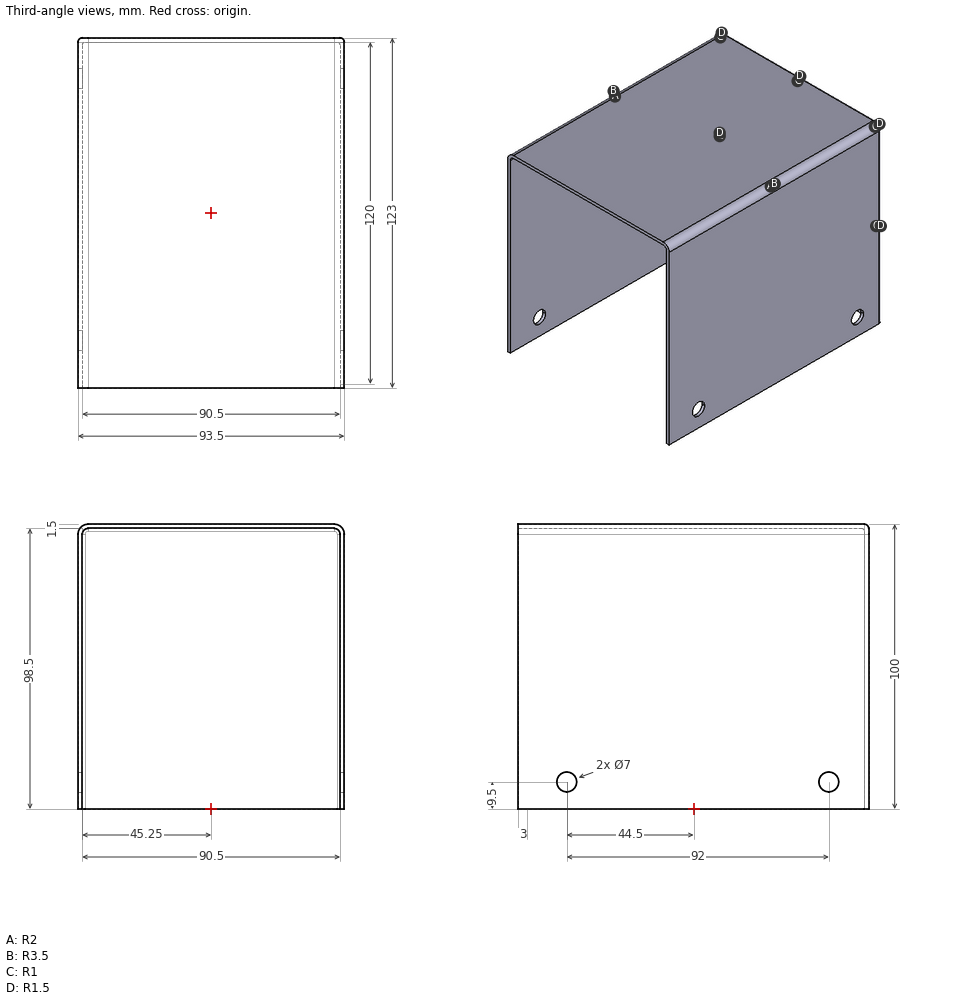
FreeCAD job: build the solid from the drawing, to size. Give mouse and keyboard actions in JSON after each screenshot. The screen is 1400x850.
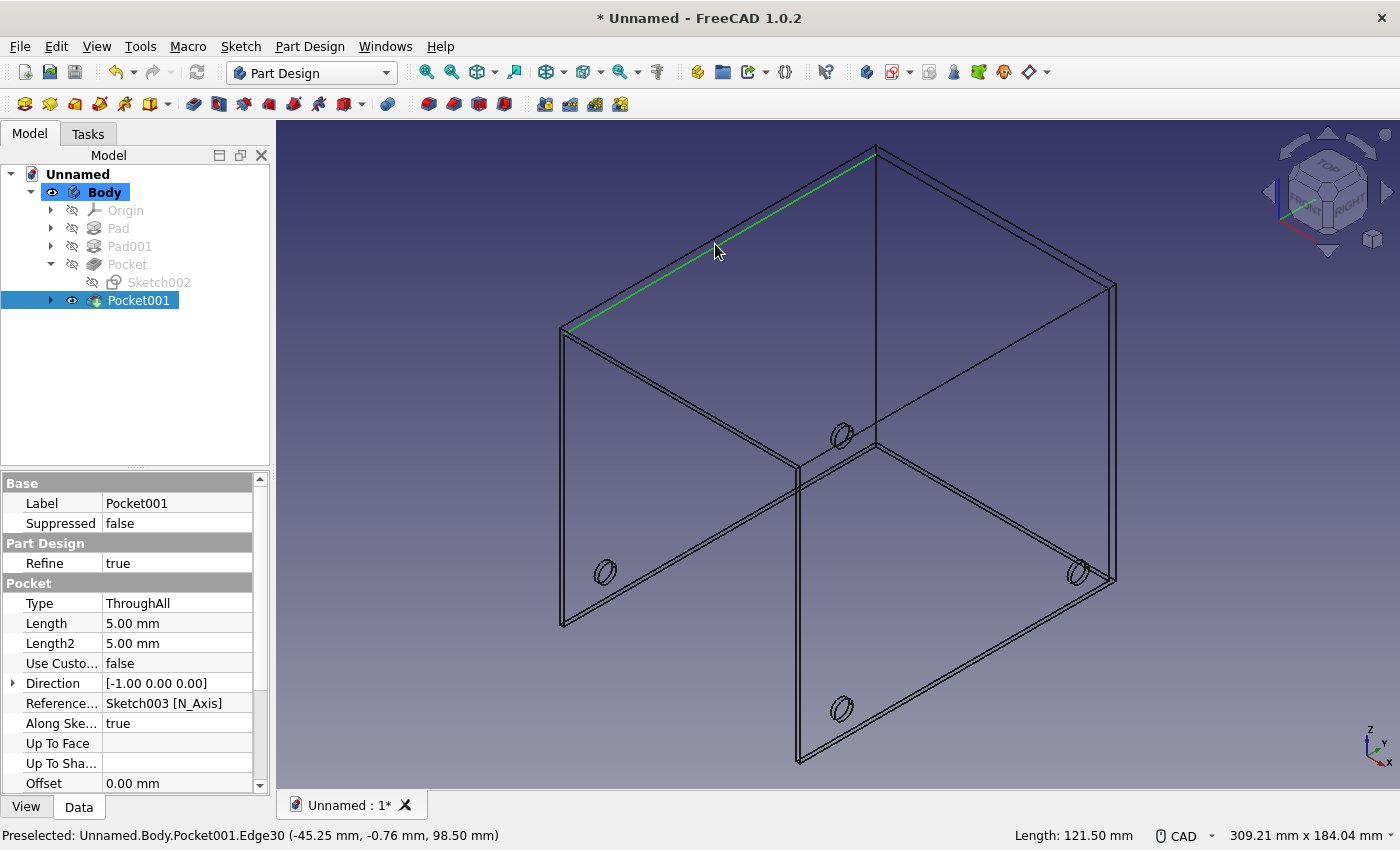
{"action": "scroll", "coordinate": [952, 378], "scroll_direction": "up", "scroll_amount": 6}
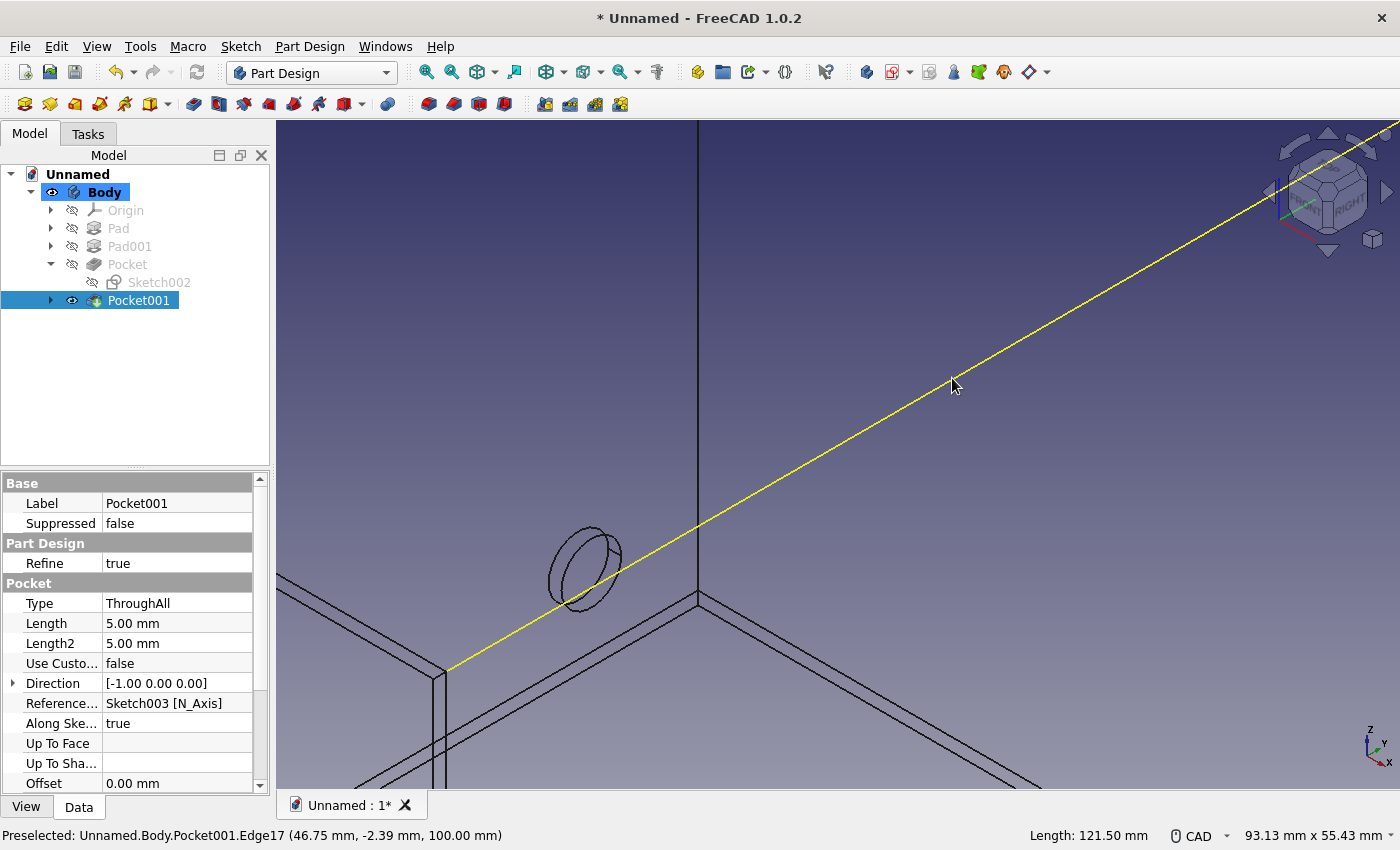
{"action": "left_click", "coordinate": [427, 72]}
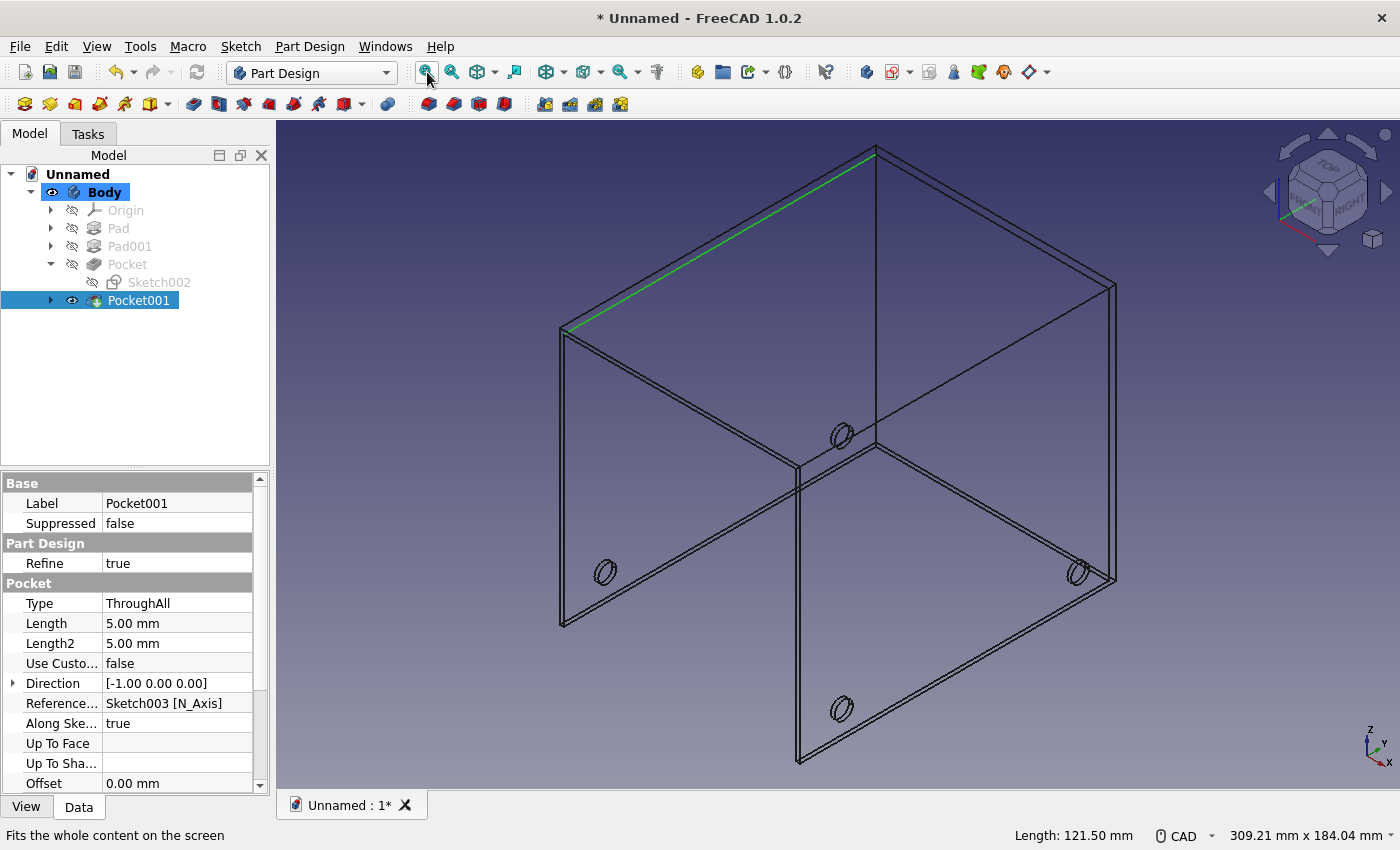
{"action": "key", "text": "2"}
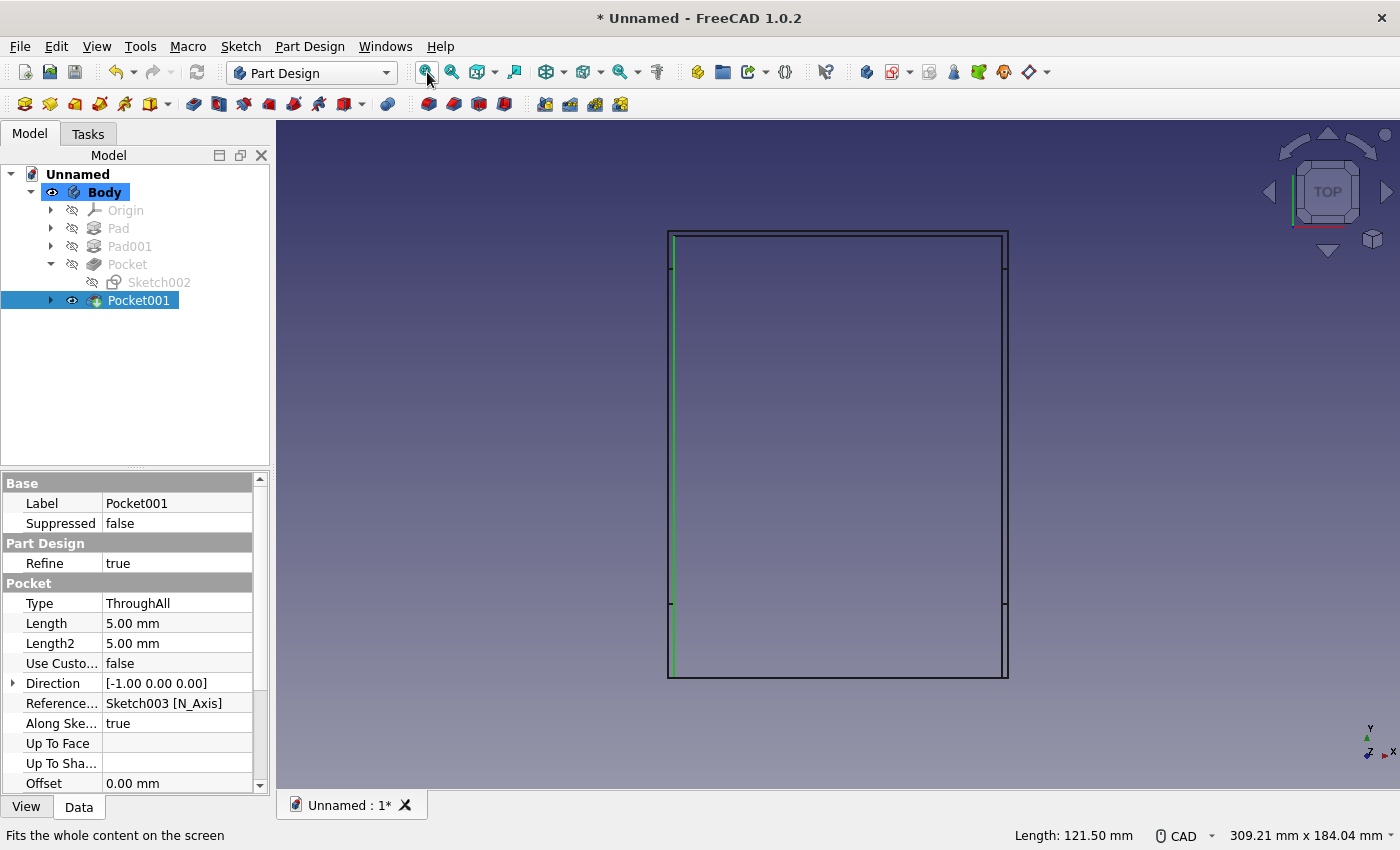
{"action": "scroll", "coordinate": [1002, 456], "scroll_direction": "up", "scroll_amount": 6}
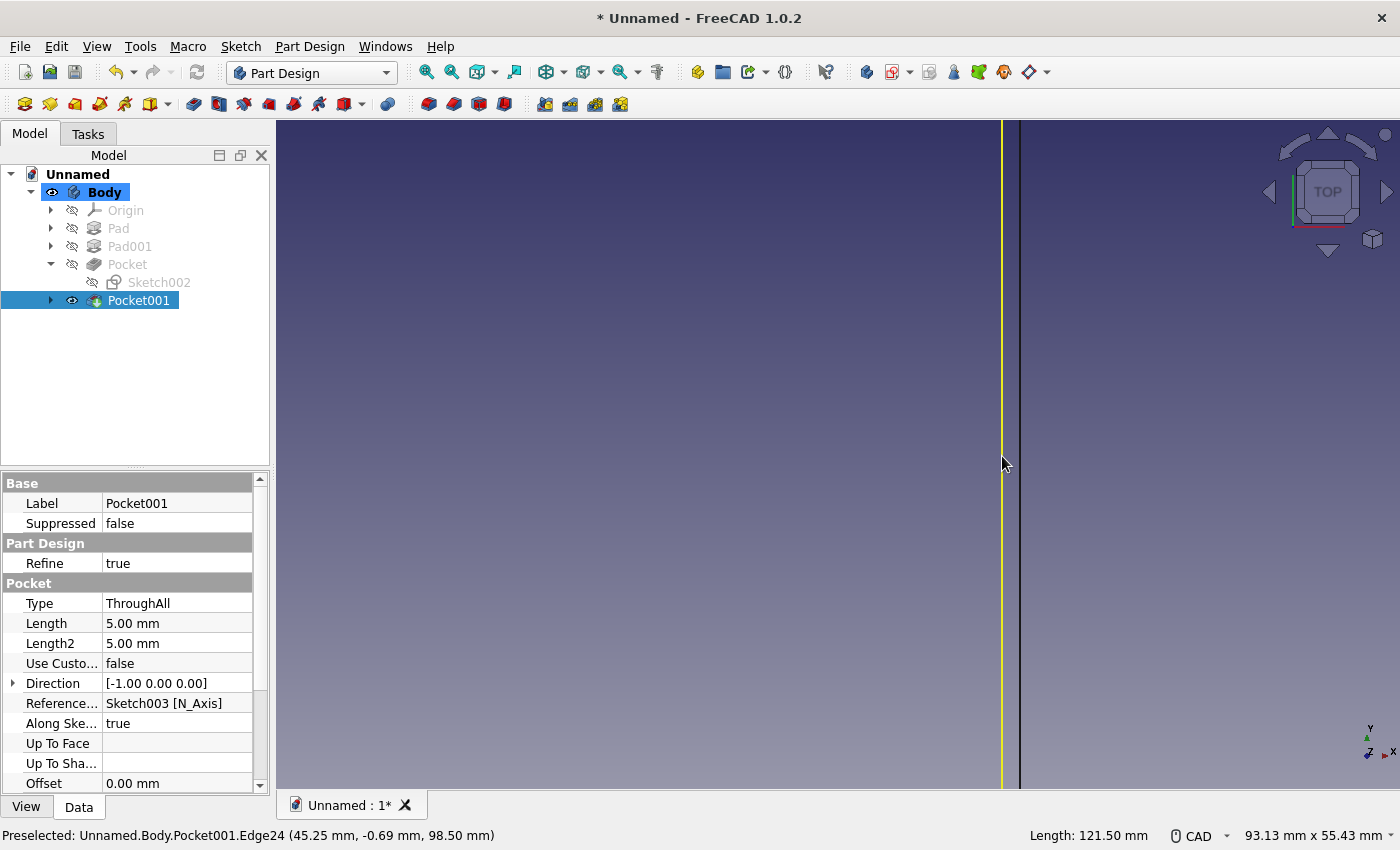
{"action": "left_click", "coordinate": [1002, 458], "text": "ctrl"}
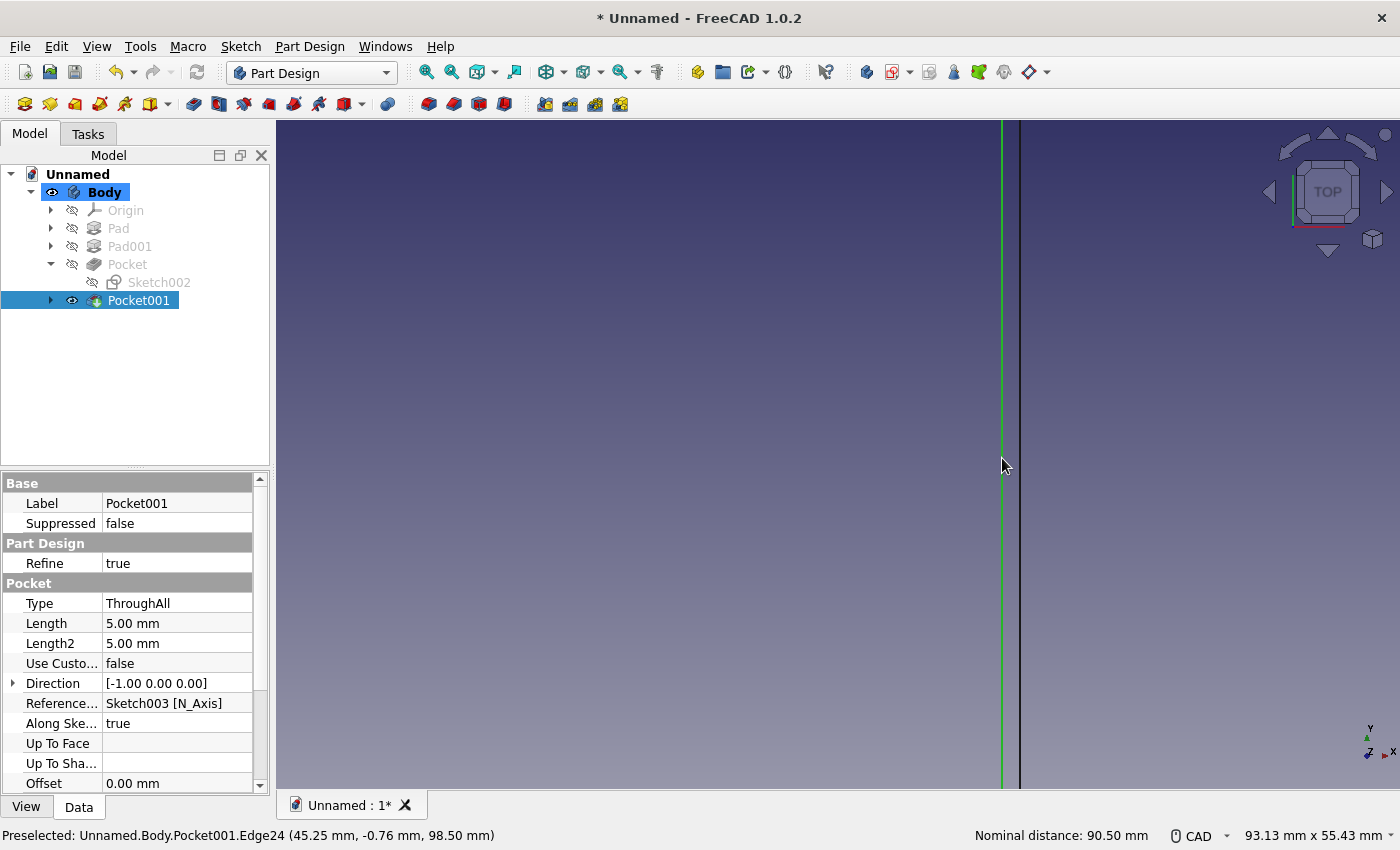
{"action": "key", "text": "v 1"}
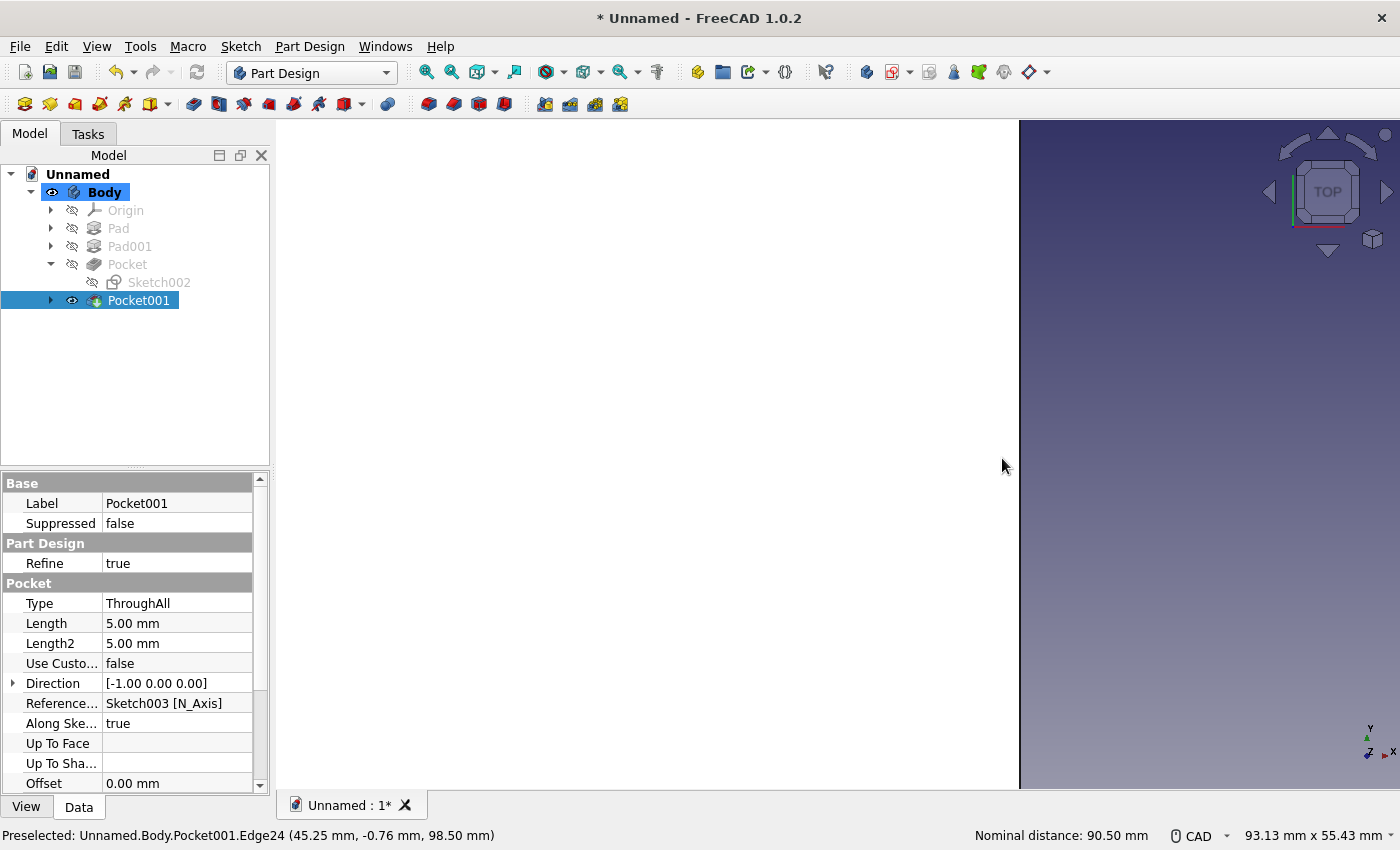
{"action": "left_click", "coordinate": [429, 104]}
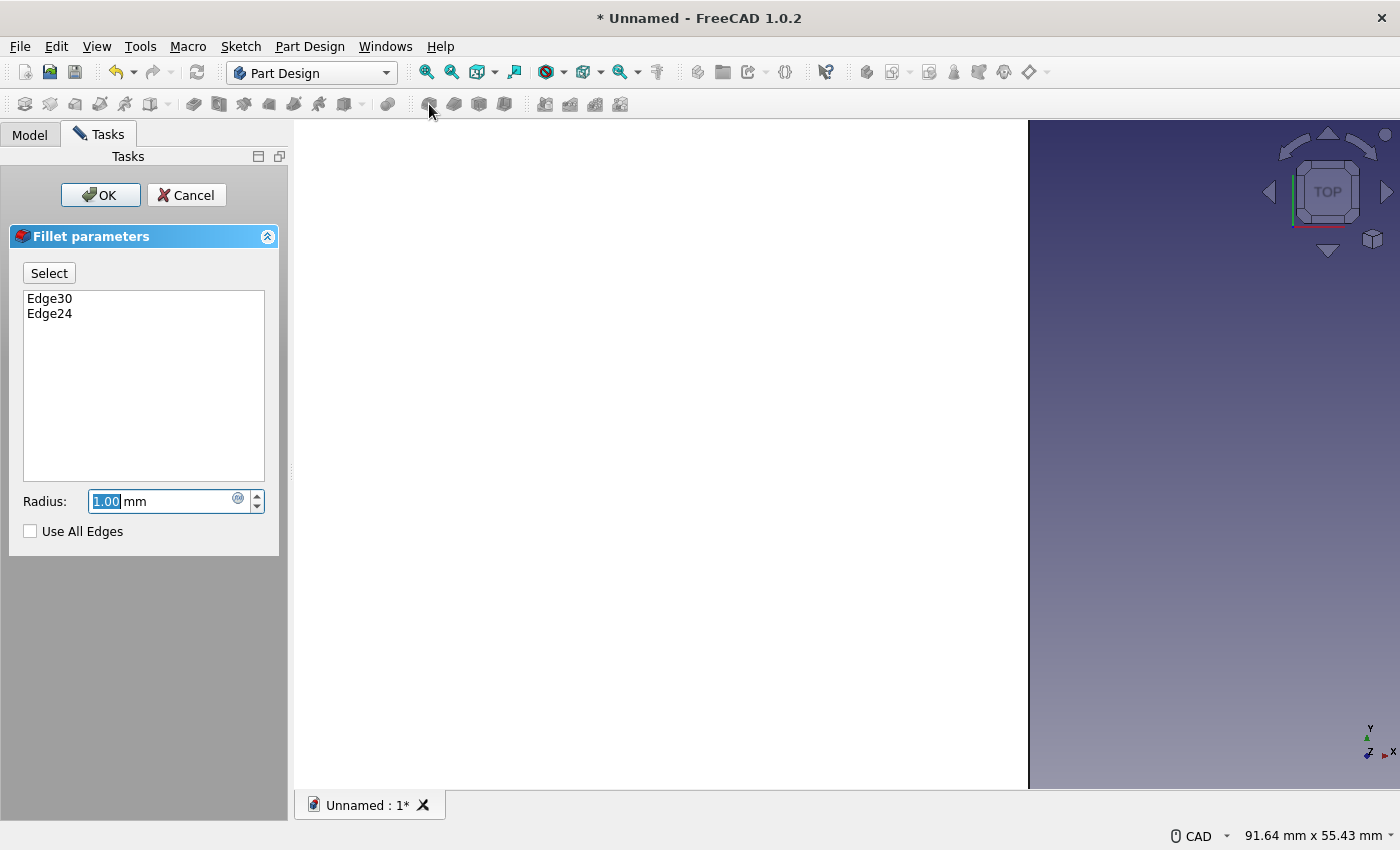
{"action": "type", "text": "2"}
{"action": "key", "text": "Tab"}